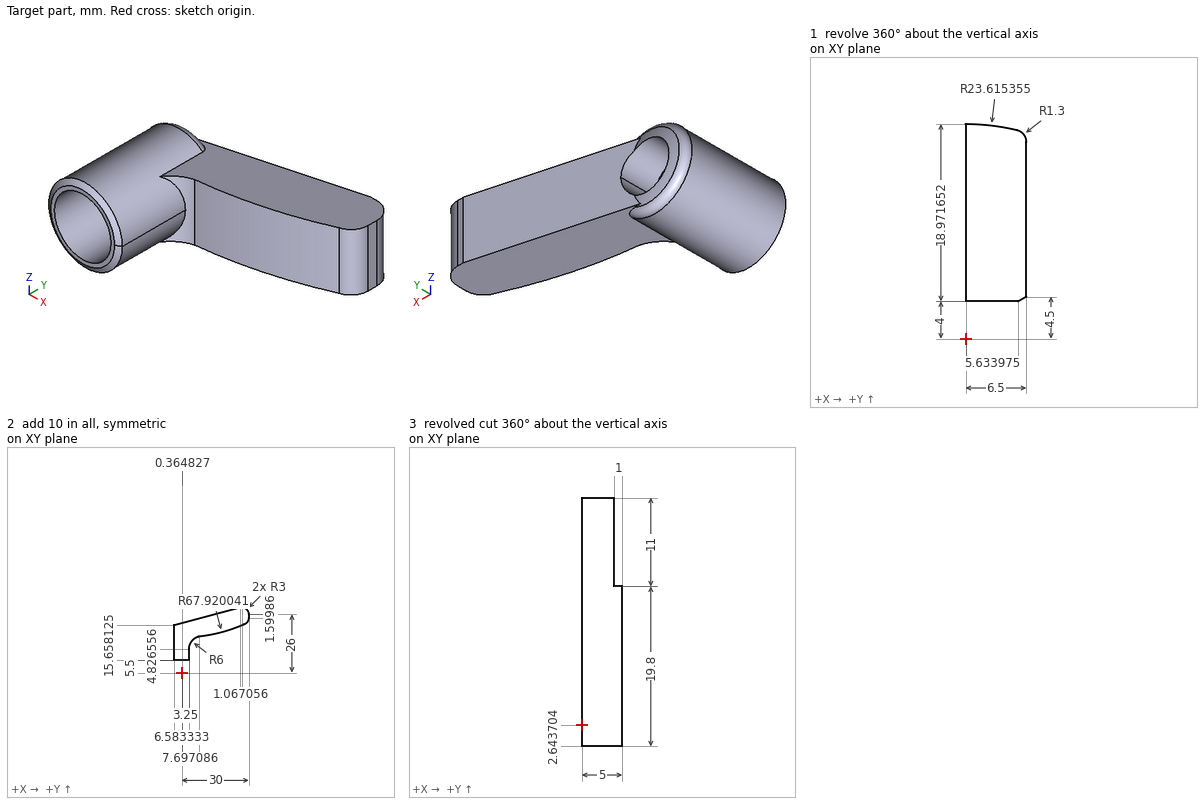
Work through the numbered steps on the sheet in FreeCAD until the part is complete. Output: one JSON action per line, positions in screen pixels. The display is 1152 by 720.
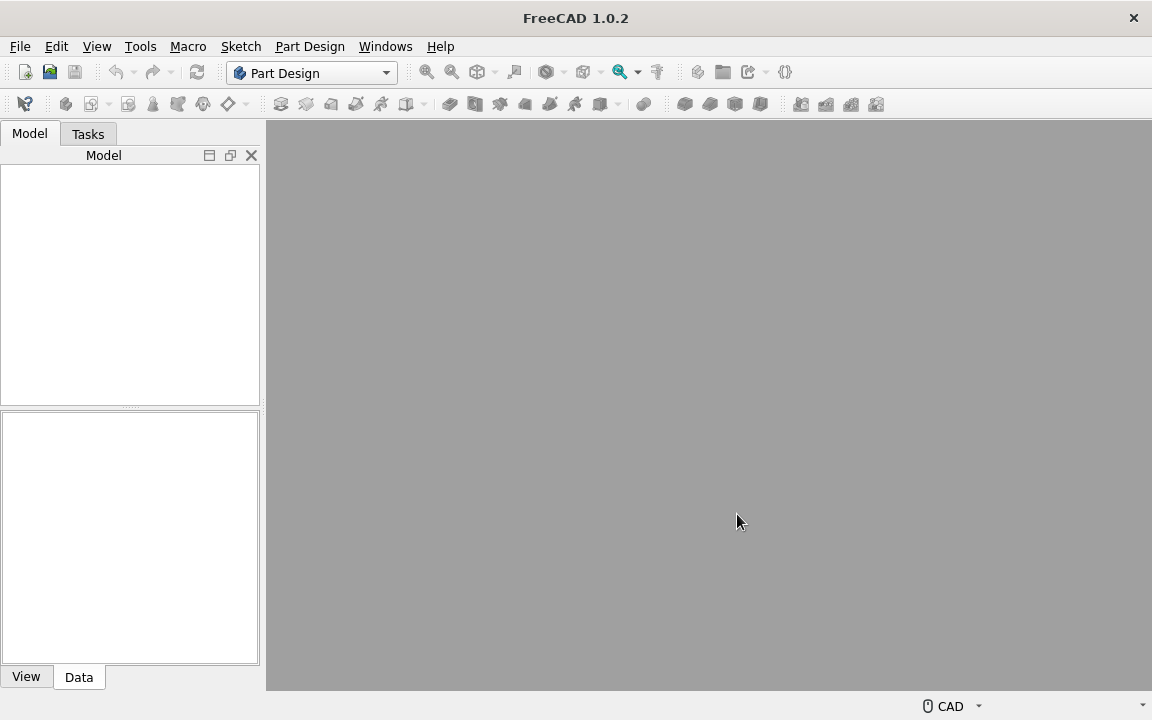
{"action": "key", "text": "ctrl+n"}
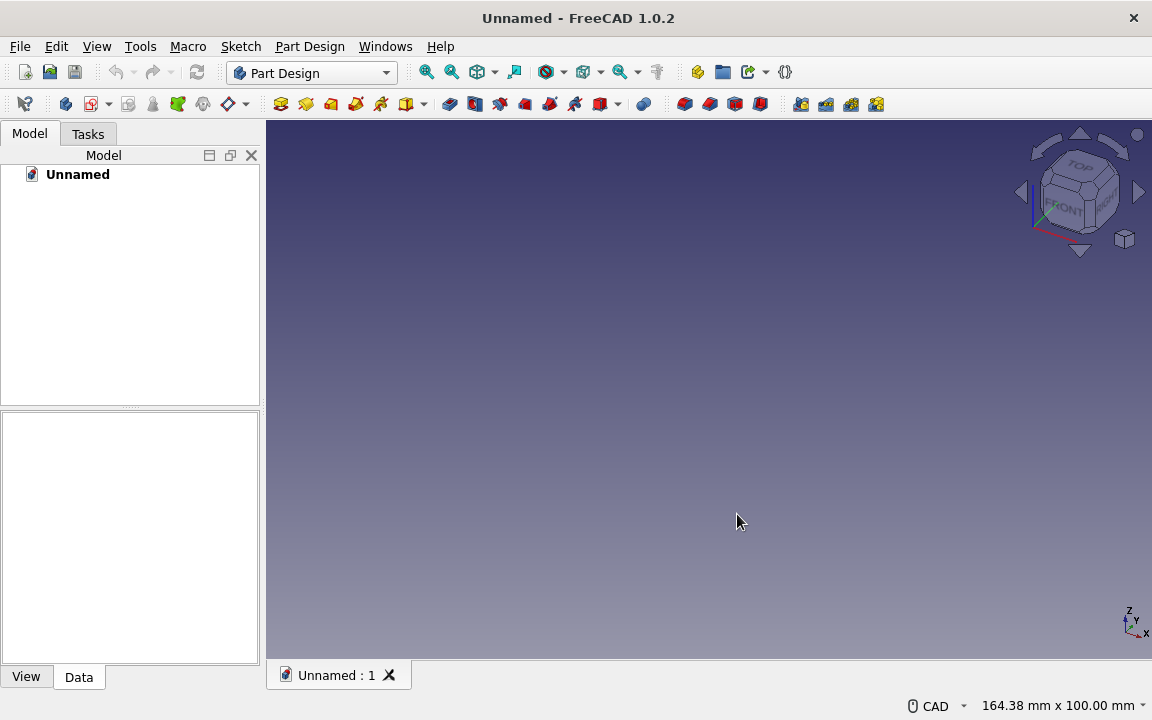
{"action": "left_click", "coordinate": [90, 104]}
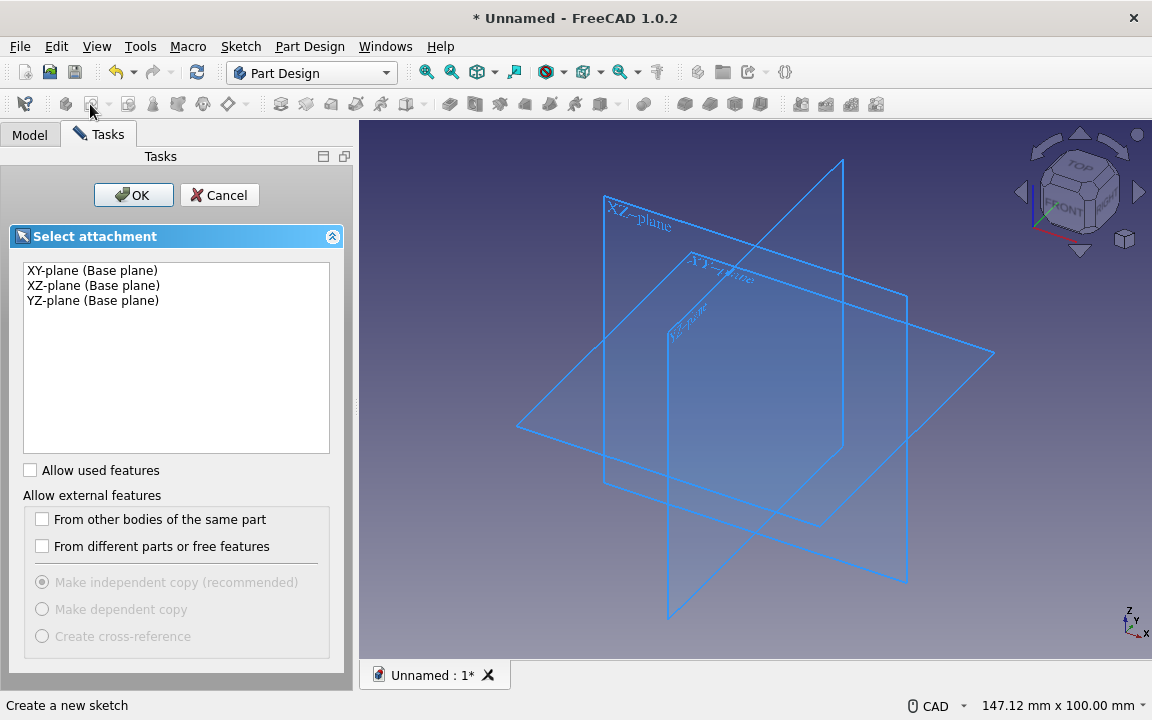
{"action": "left_click", "coordinate": [84, 270]}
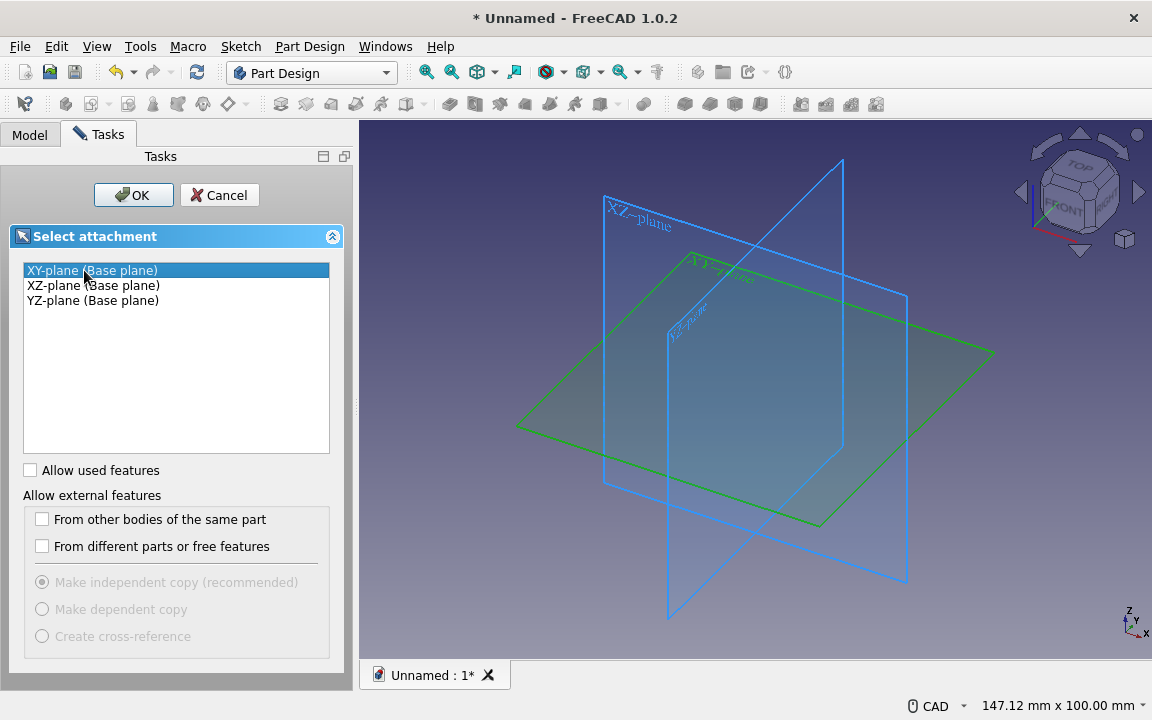
{"action": "left_click", "coordinate": [134, 195]}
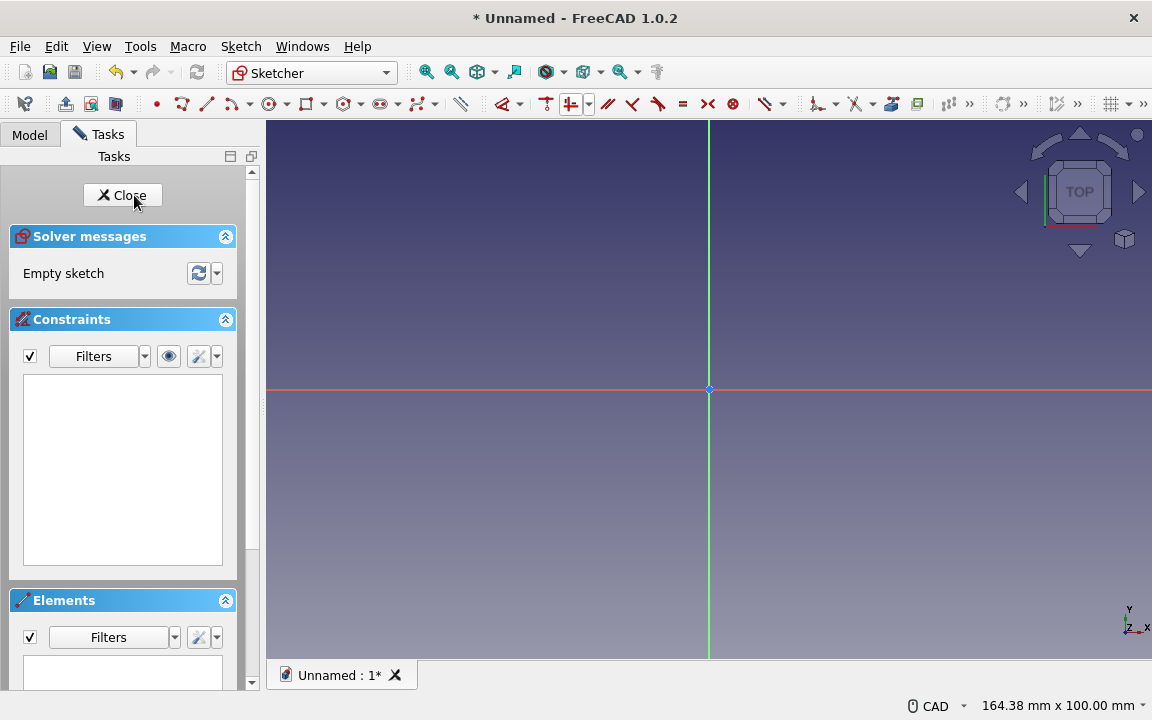
{"action": "scroll", "coordinate": [777, 292], "scroll_direction": "up", "scroll_amount": 5}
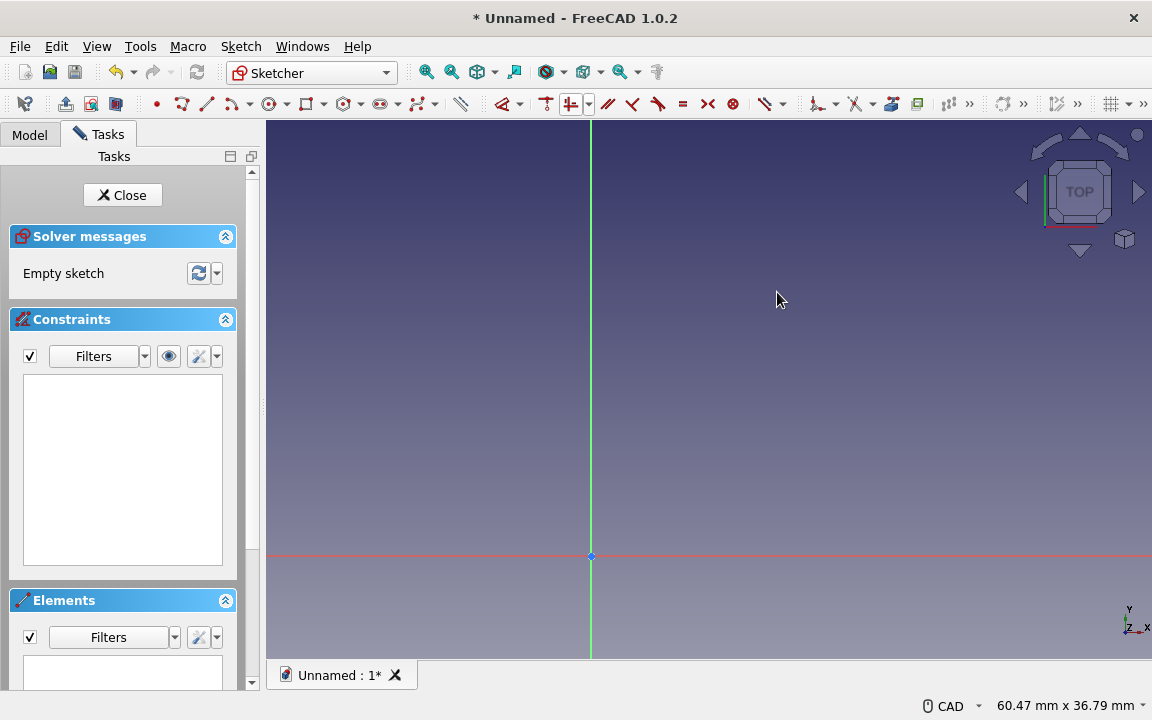
{"action": "left_click", "coordinate": [182, 104]}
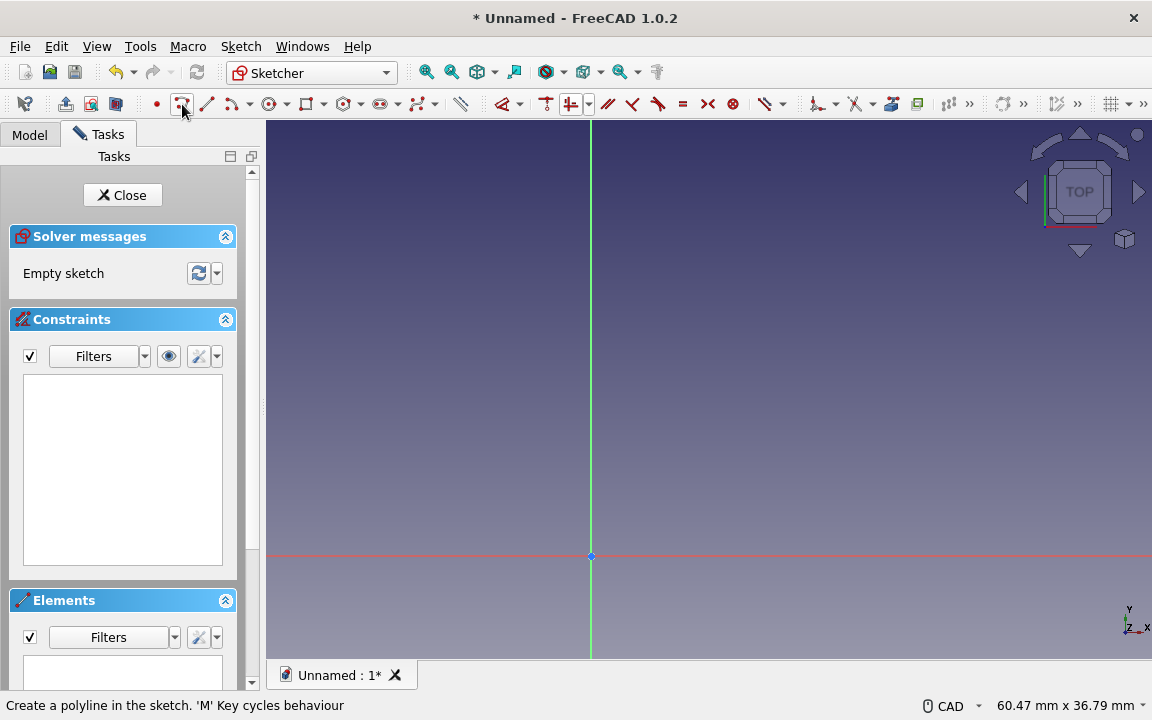
{"action": "left_click", "coordinate": [591, 220]}
{"action": "left_click", "coordinate": [600, 498]}
{"action": "left_click", "coordinate": [674, 498]}
{"action": "left_click", "coordinate": [686, 491]}
{"action": "left_click", "coordinate": [686, 248]}
{"action": "right_click", "coordinate": [686, 248]}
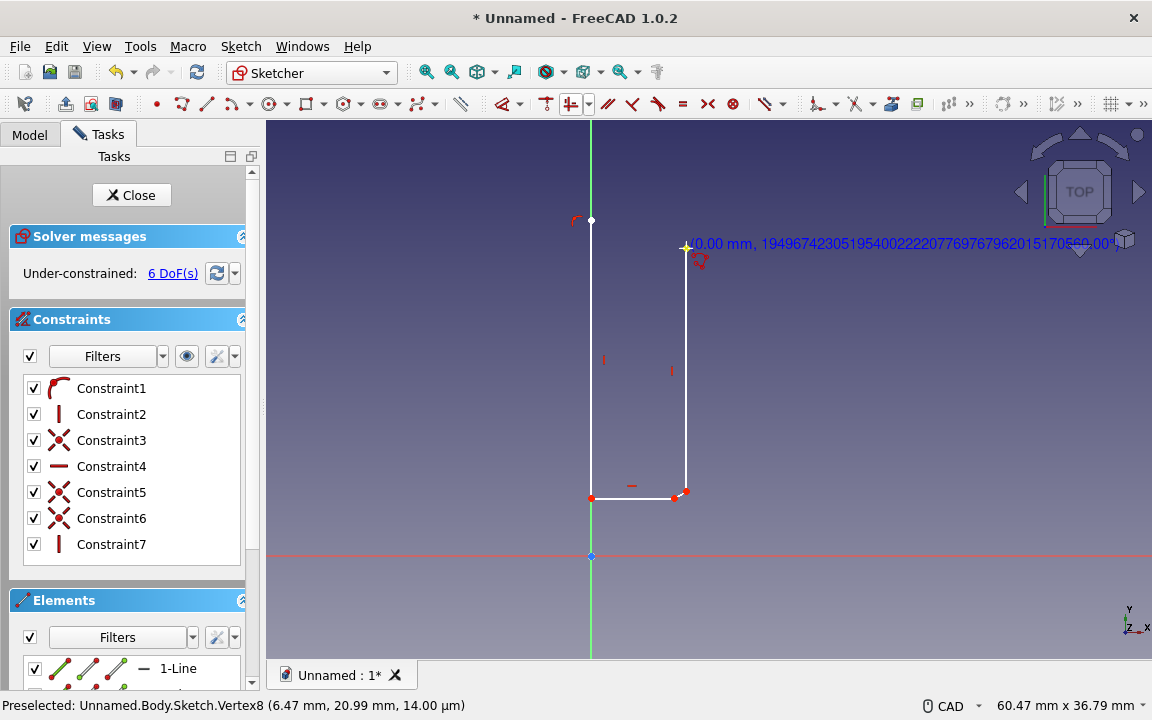
{"action": "key", "text": "g 3 a"}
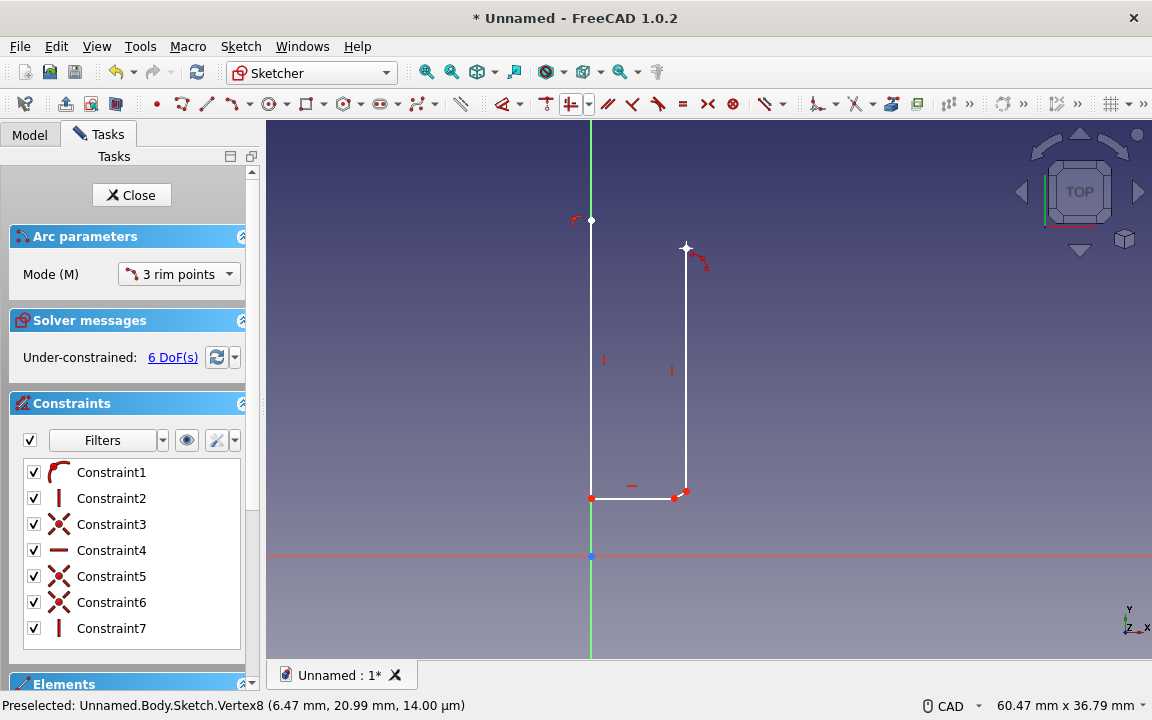
{"action": "left_click", "coordinate": [686, 249]}
{"action": "left_click", "coordinate": [672, 229]}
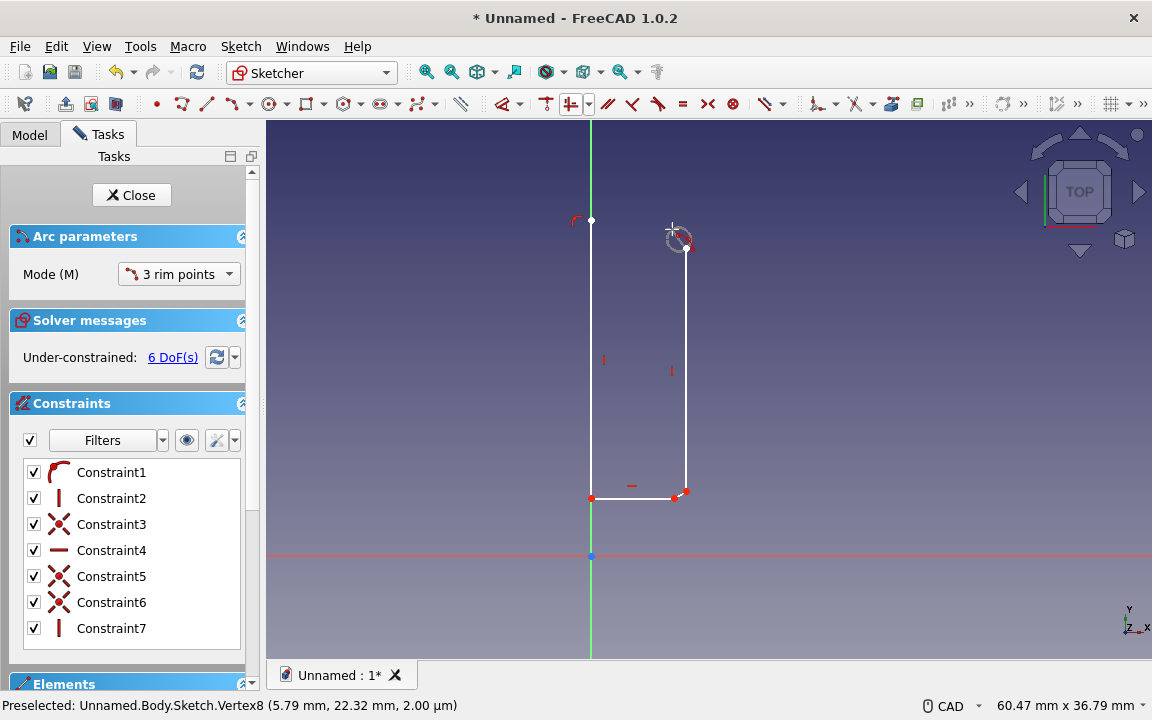
{"action": "scroll", "coordinate": [682, 236], "scroll_direction": "up", "scroll_amount": 7}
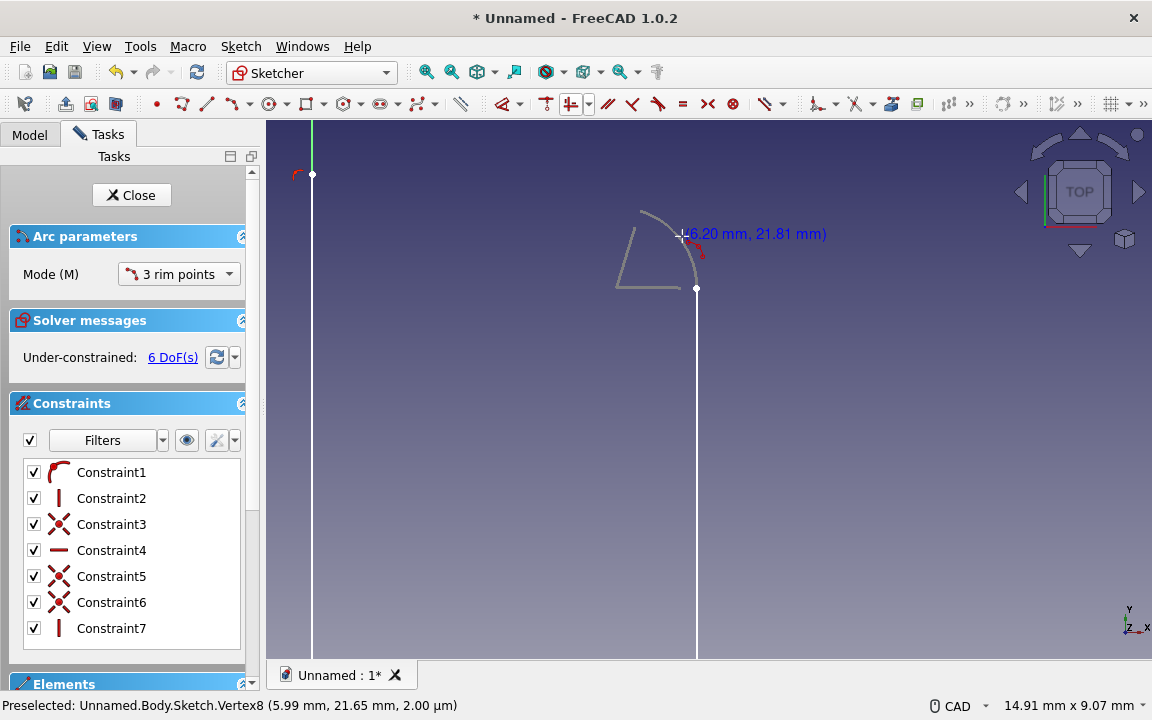
{"action": "left_click", "coordinate": [682, 236]}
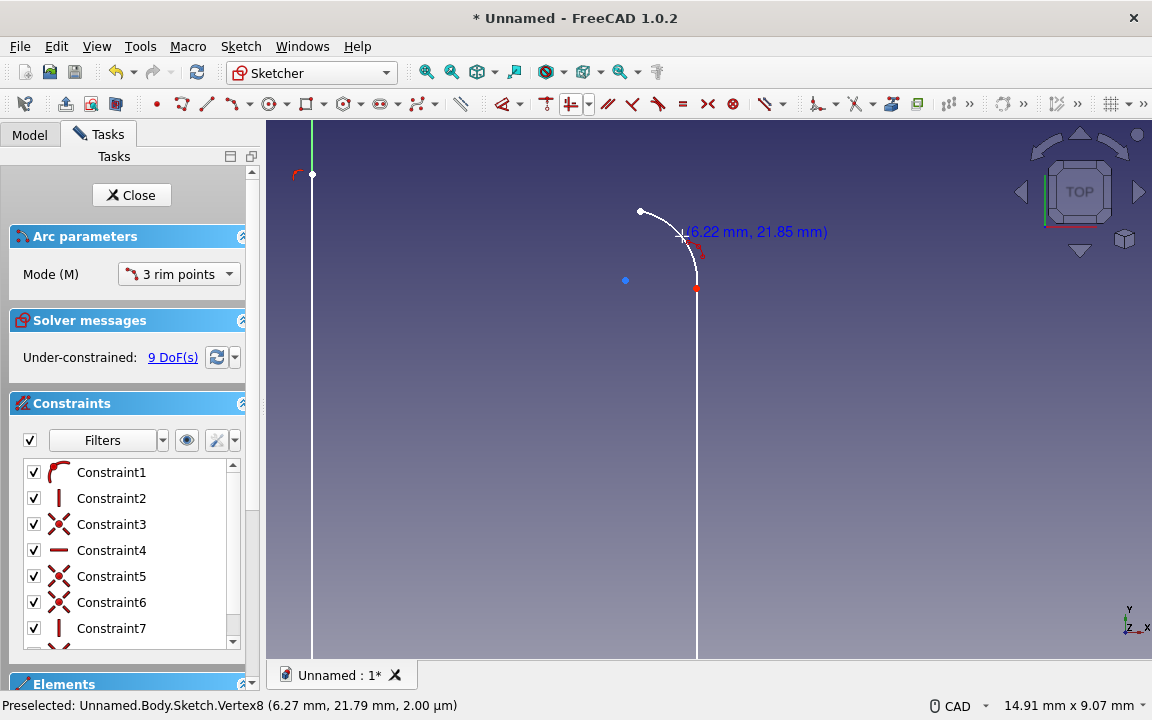
{"action": "scroll", "coordinate": [685, 238], "scroll_direction": "down", "scroll_amount": 7}